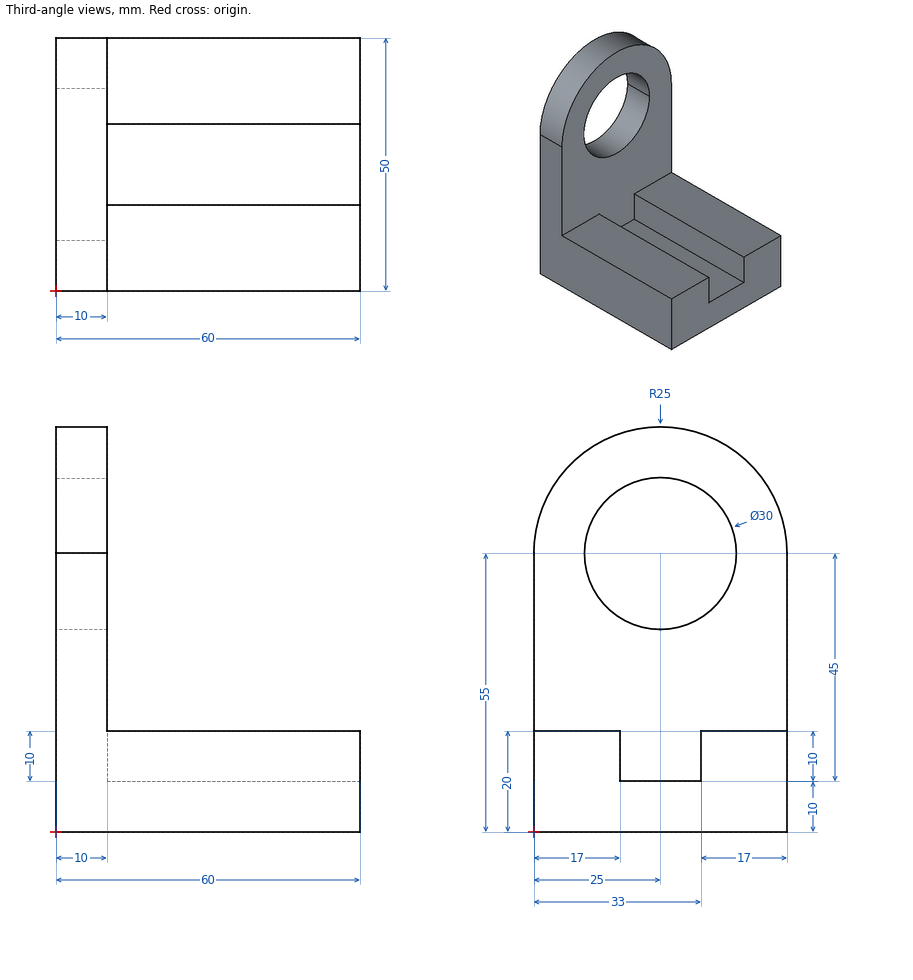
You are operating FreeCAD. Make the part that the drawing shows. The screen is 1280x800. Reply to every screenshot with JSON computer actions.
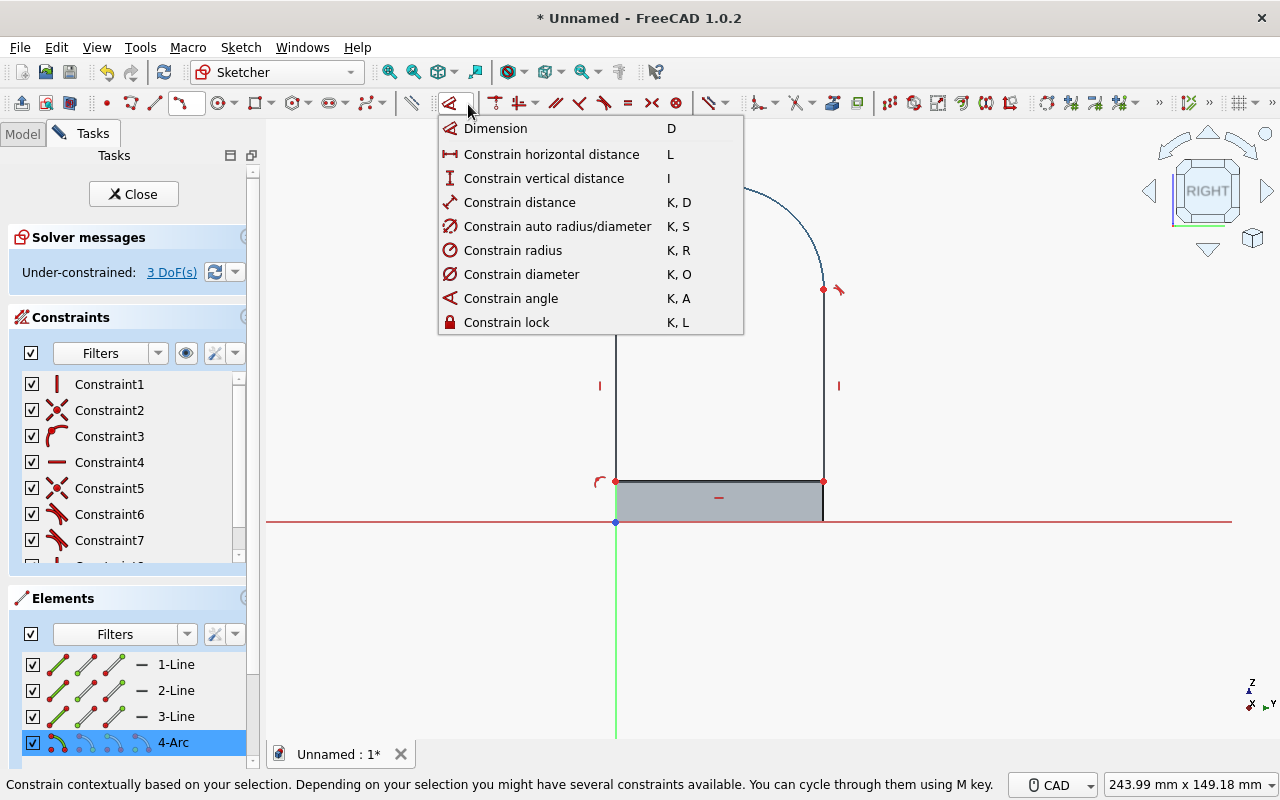
{"action": "left_click", "coordinate": [591, 250]}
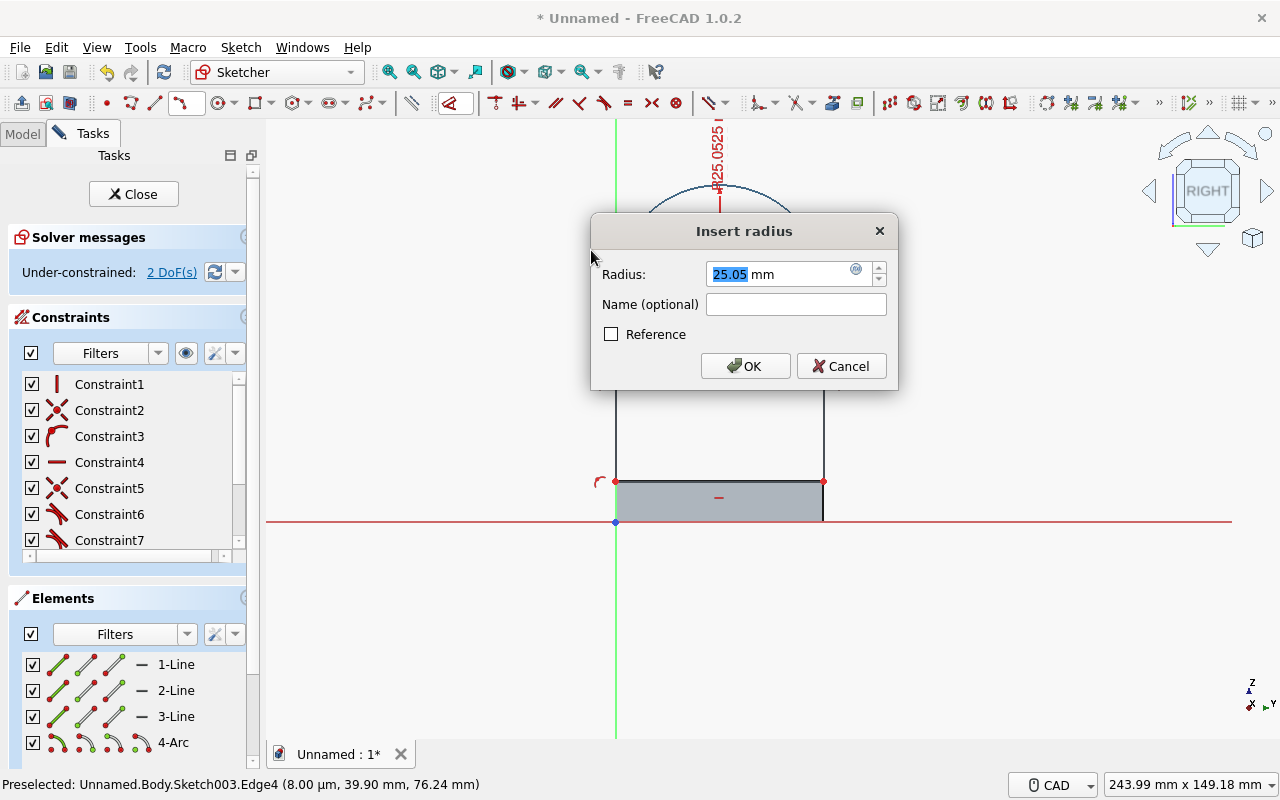
{"action": "type", "text": "25"}
{"action": "key", "text": "Return"}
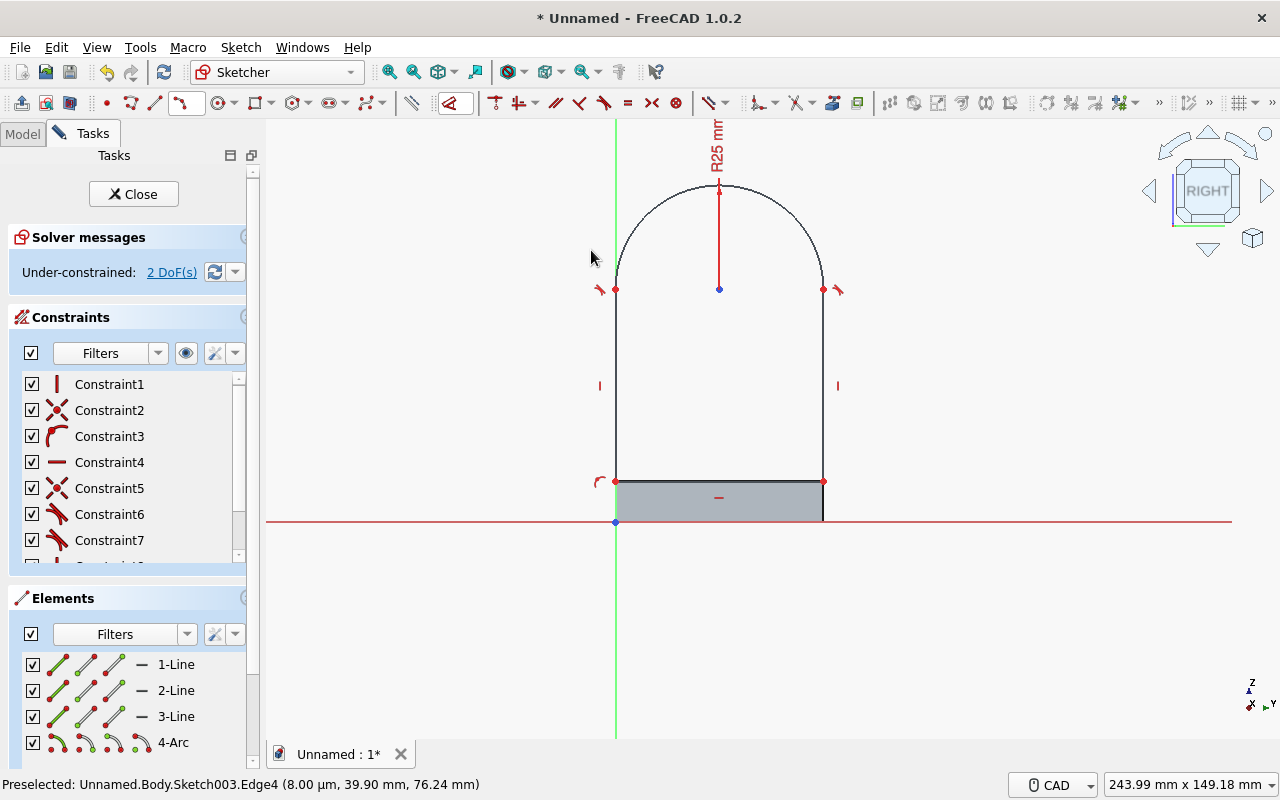
{"action": "left_click", "coordinate": [823, 347]}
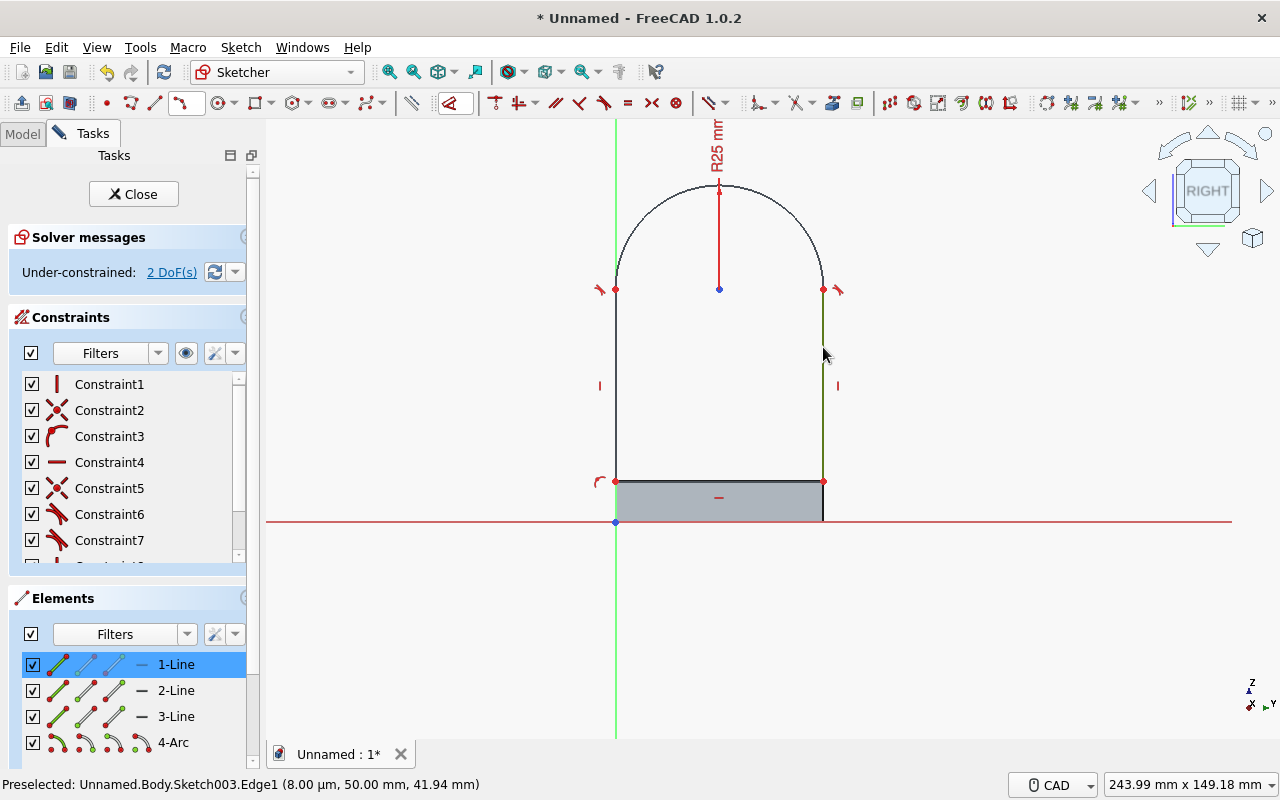
{"action": "left_click", "coordinate": [468, 104]}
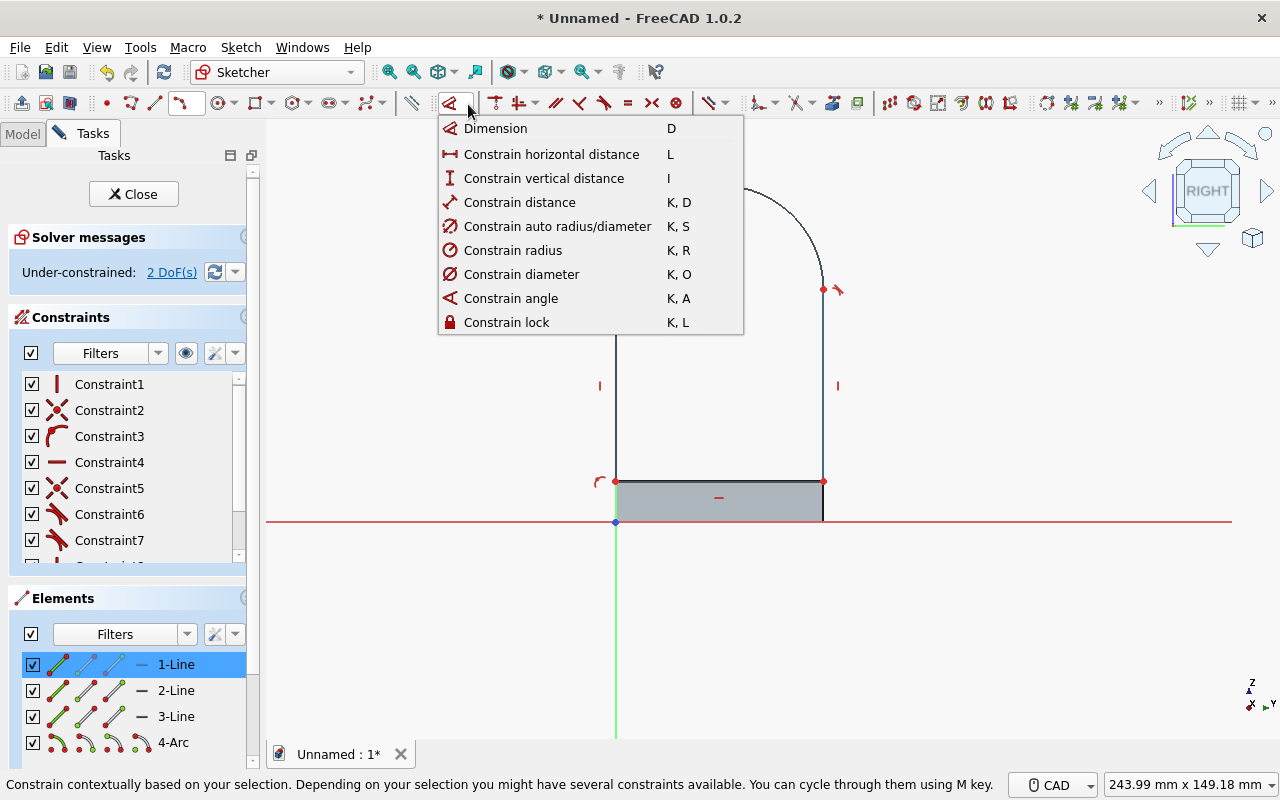
{"action": "left_click", "coordinate": [591, 178]}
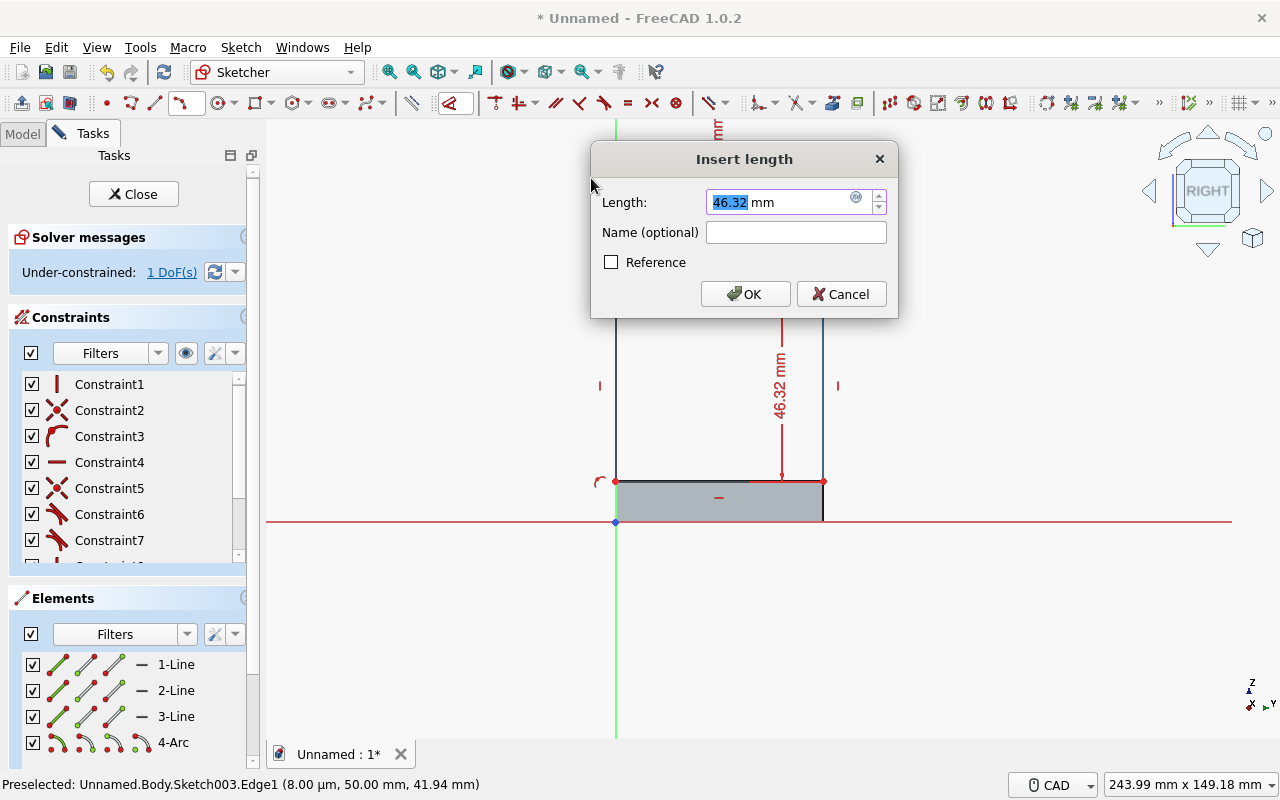
{"action": "type", "text": "45"}
{"action": "key", "text": "Return"}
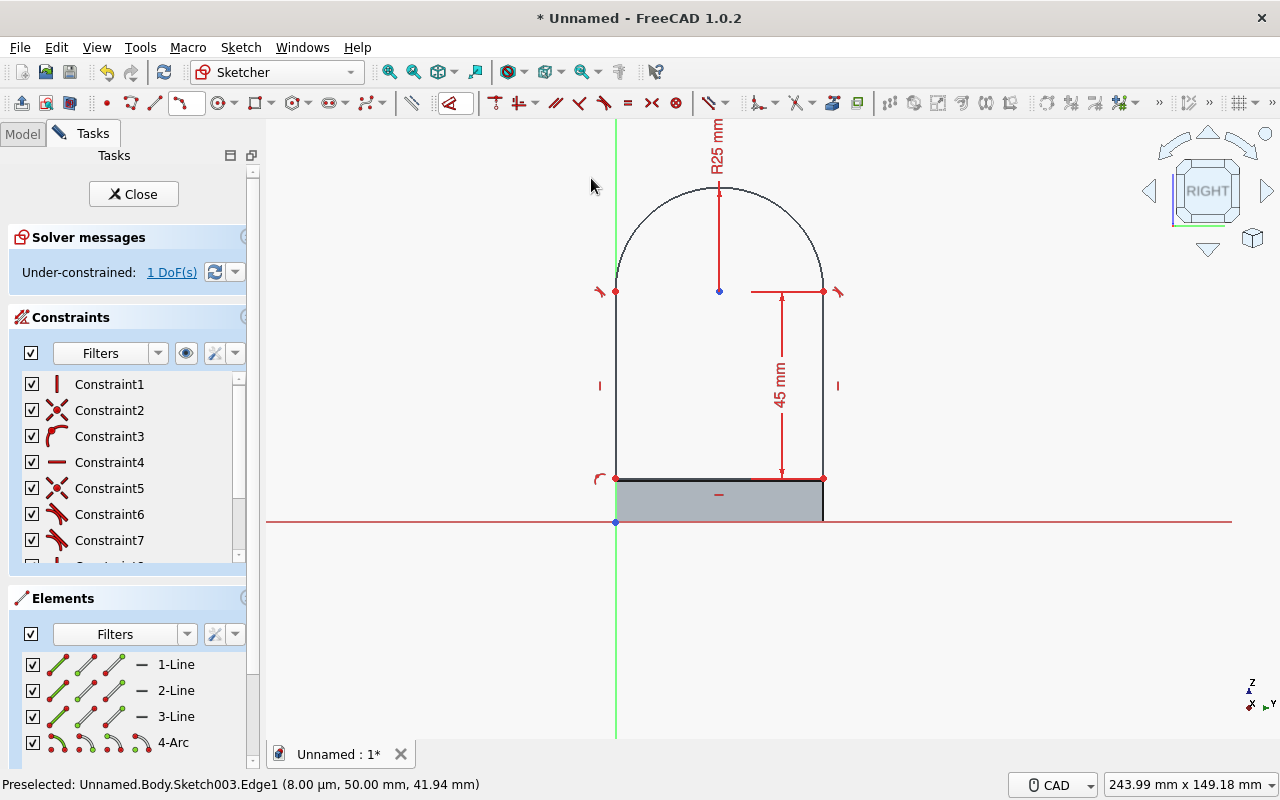
{"action": "left_click", "coordinate": [823, 292]}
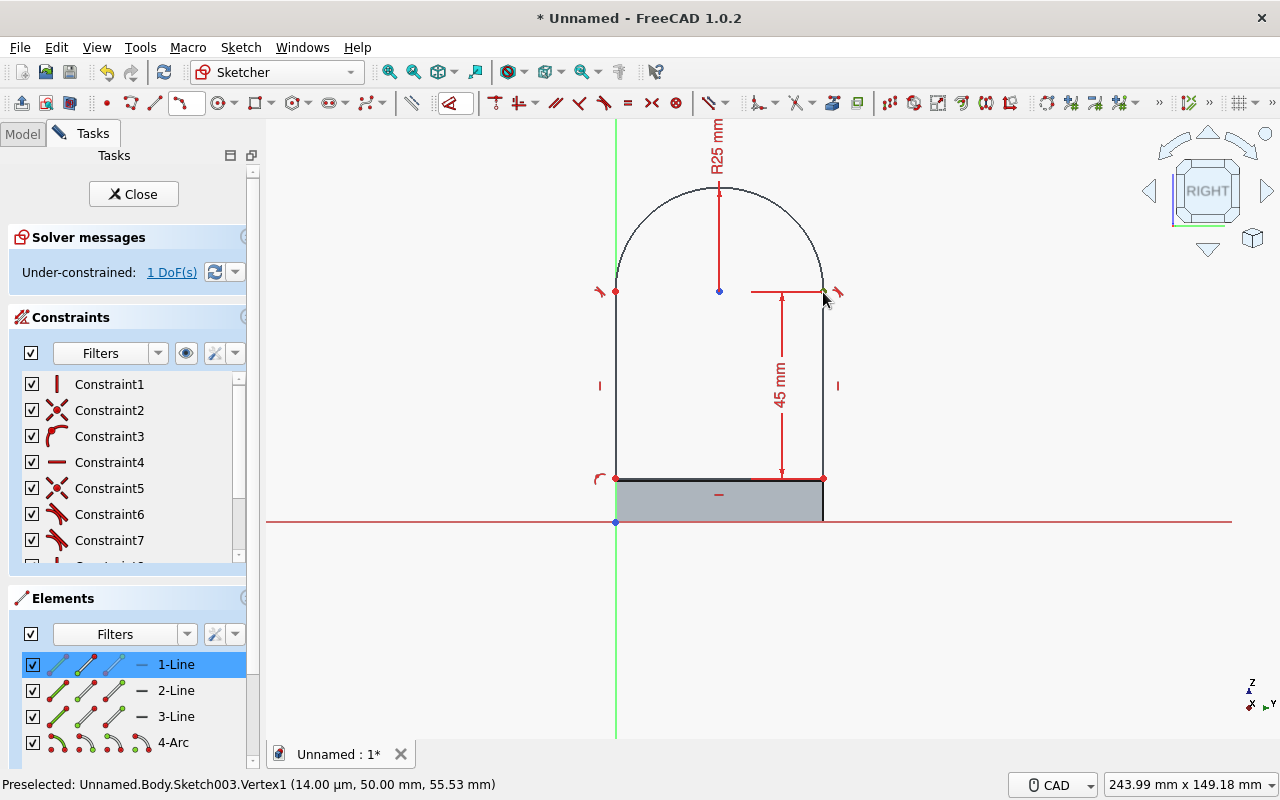
{"action": "key", "text": "i"}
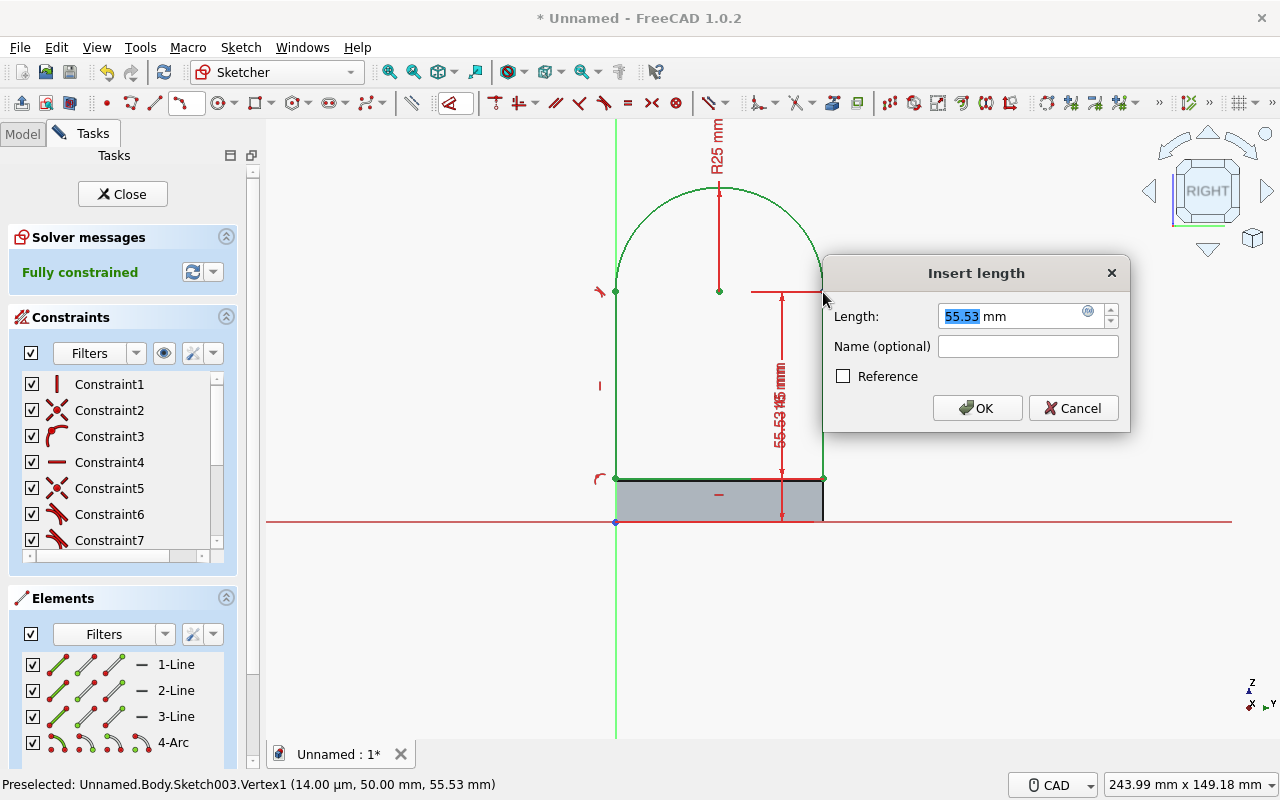
{"action": "type", "text": "55"}
{"action": "key", "text": "Return"}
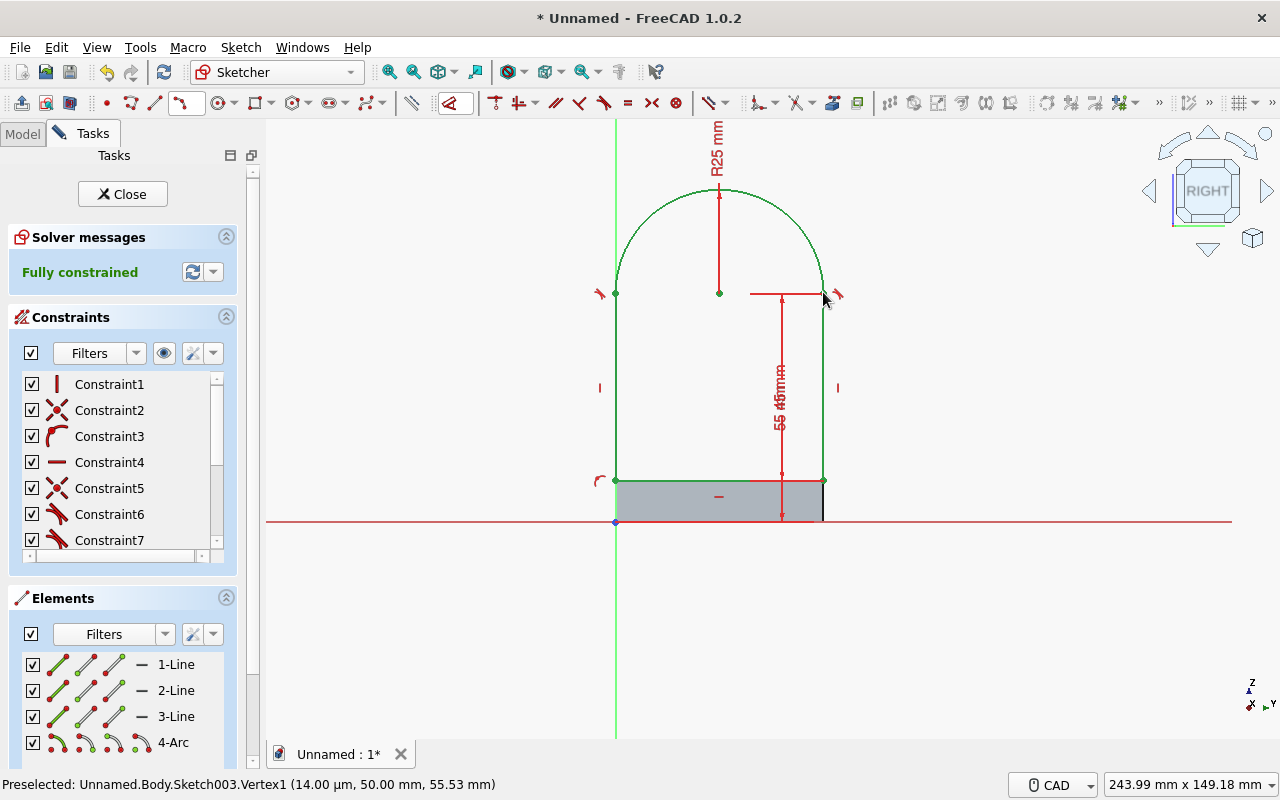
{"action": "left_click", "coordinate": [123, 194]}